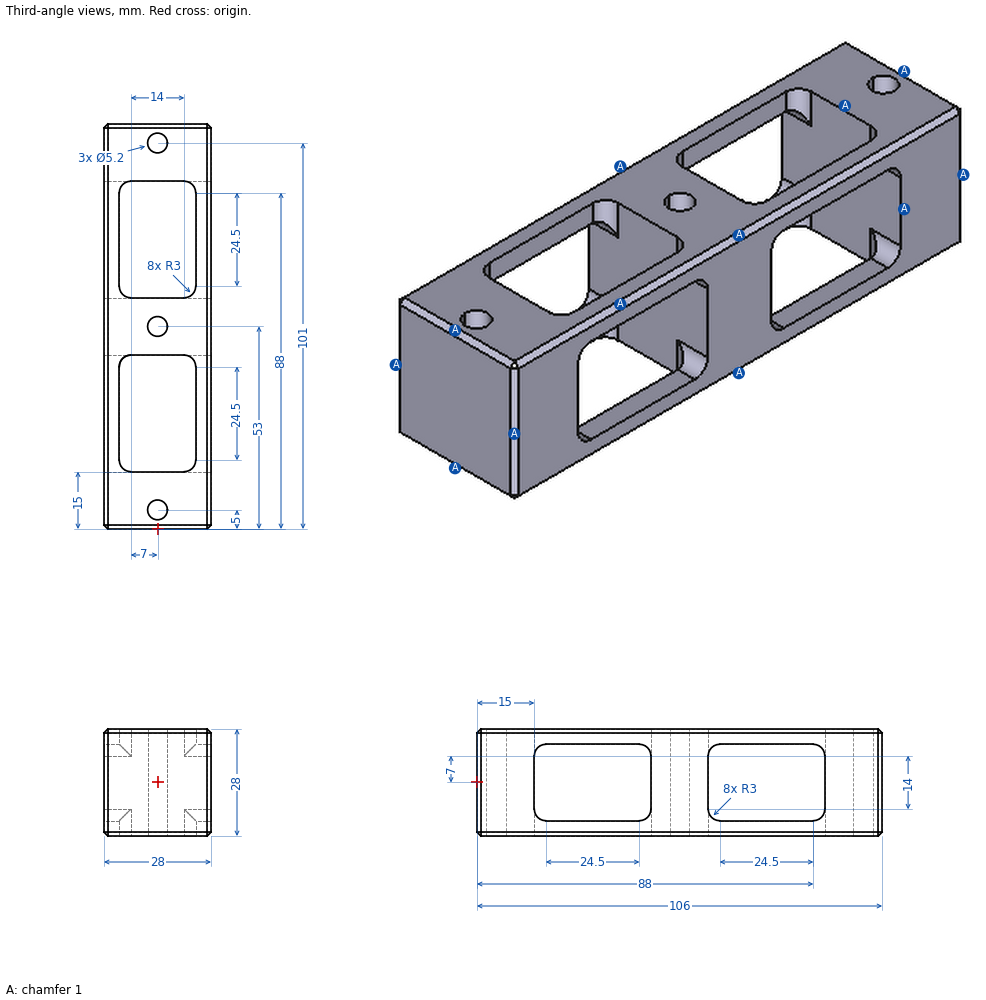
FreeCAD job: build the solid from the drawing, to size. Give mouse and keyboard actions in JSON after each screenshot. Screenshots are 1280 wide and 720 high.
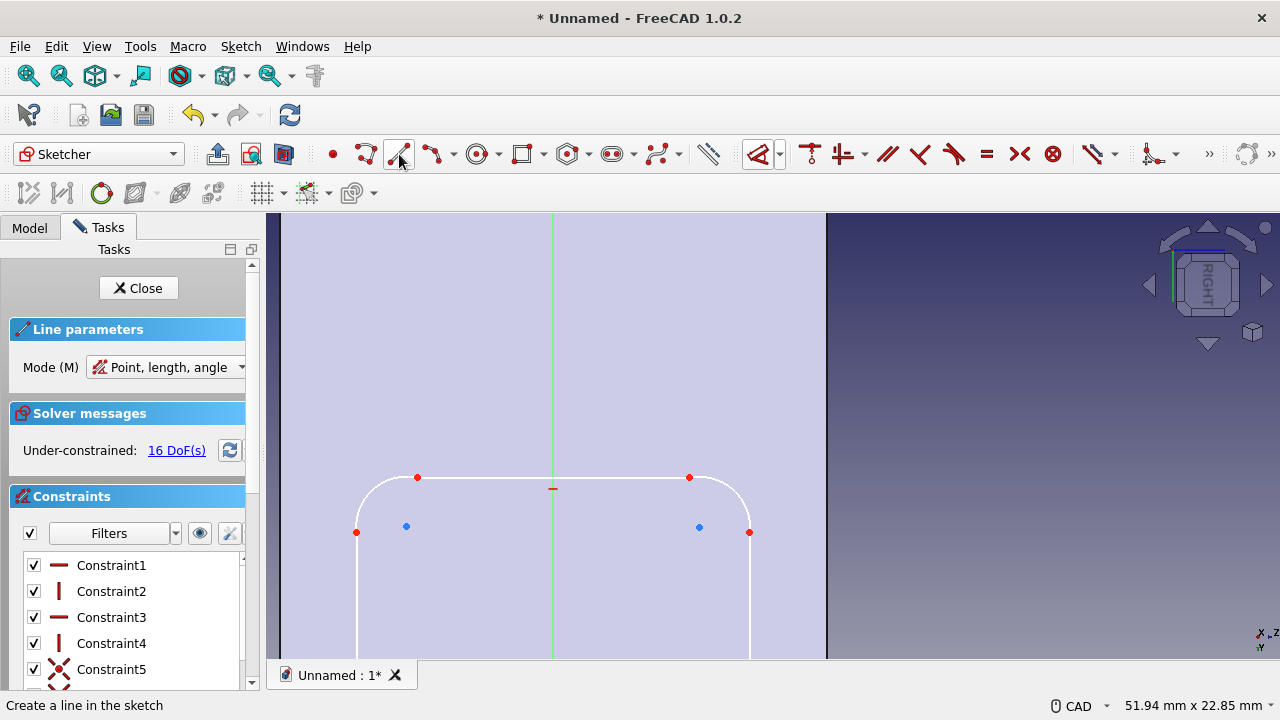
{"action": "scroll", "coordinate": [734, 487], "scroll_direction": "down", "scroll_amount": 9}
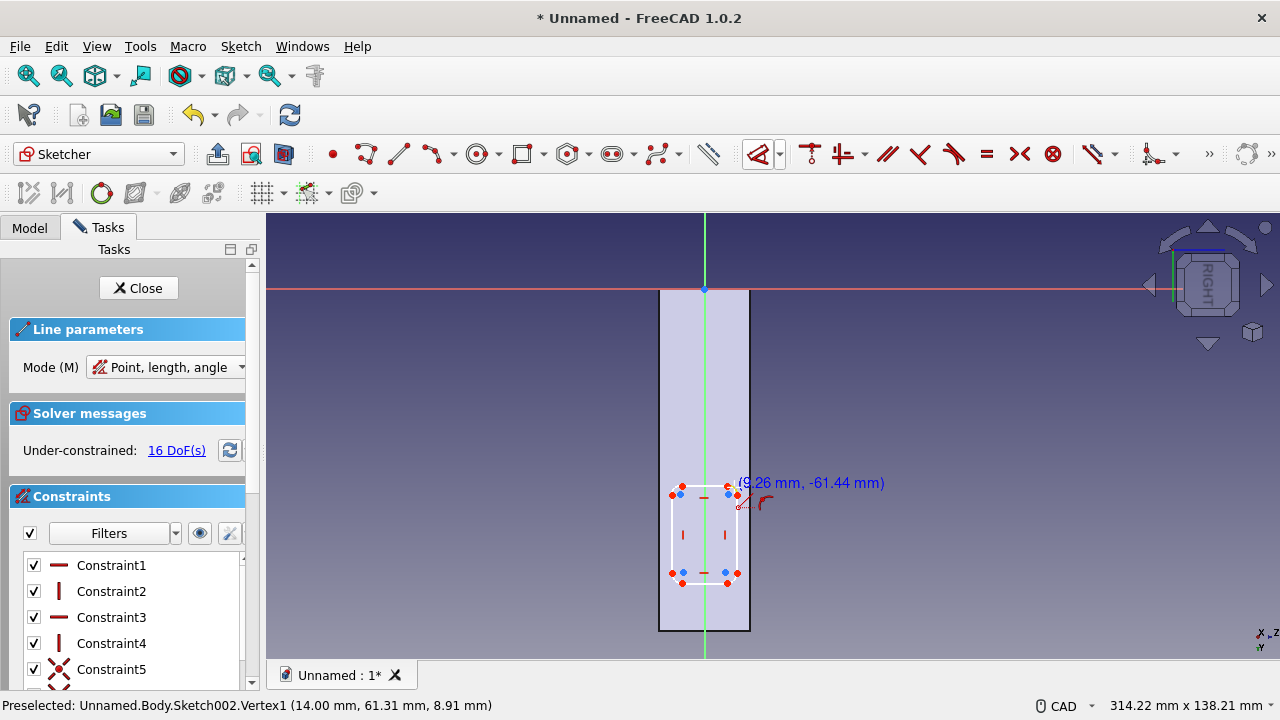
{"action": "left_click", "coordinate": [727, 338]}
{"action": "left_click", "coordinate": [682, 338]}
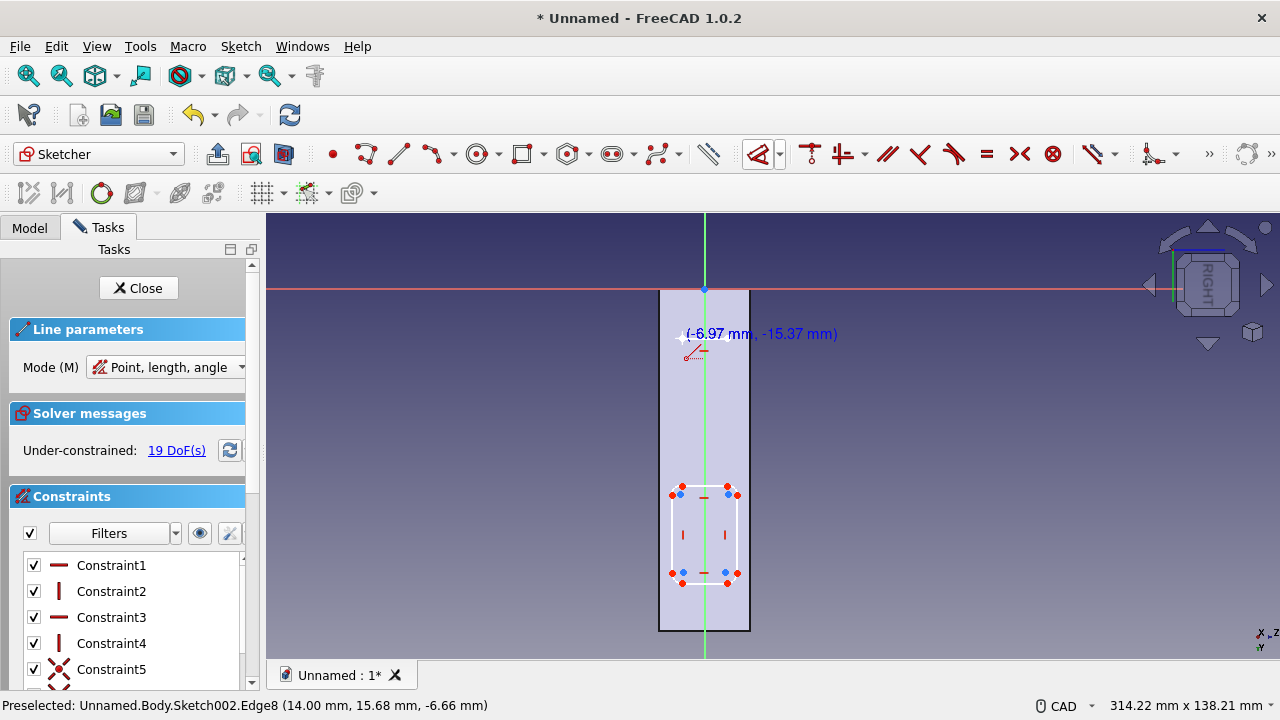
{"action": "left_click", "coordinate": [672, 347]}
{"action": "left_click", "coordinate": [672, 427]}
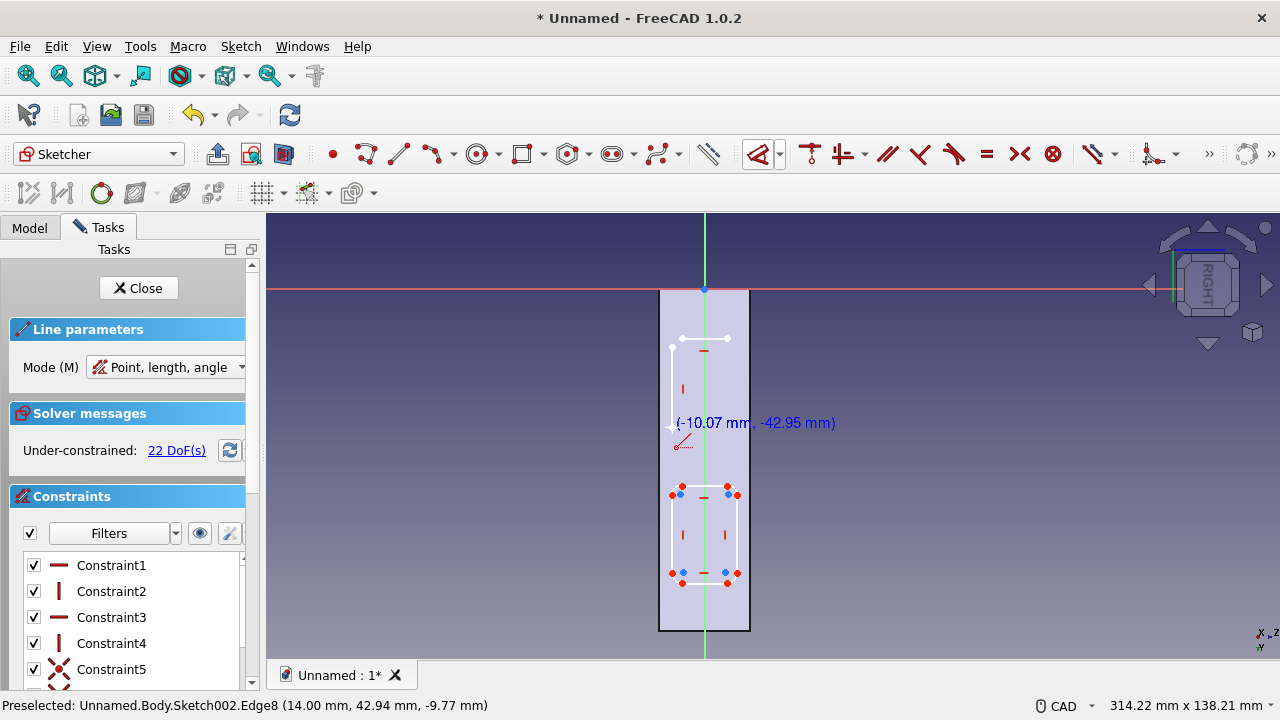
{"action": "left_click", "coordinate": [682, 436]}
{"action": "left_click", "coordinate": [727, 436]}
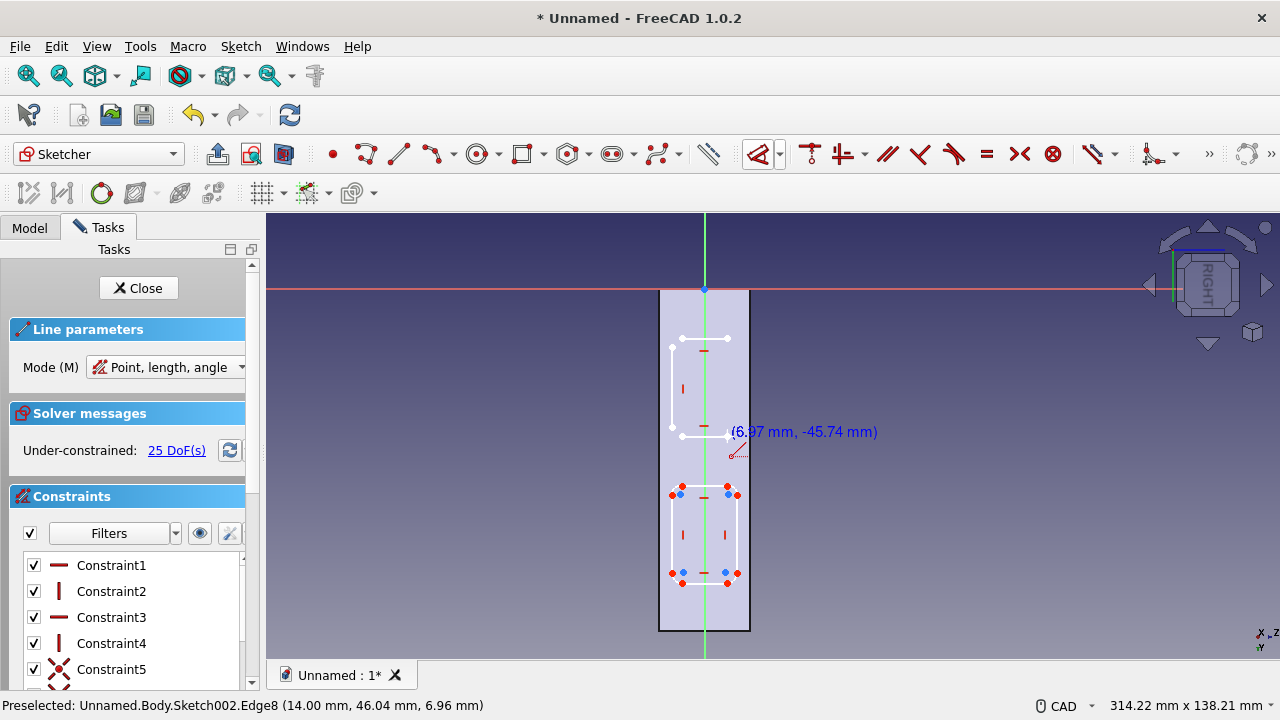
{"action": "left_click", "coordinate": [737, 427]}
{"action": "left_click", "coordinate": [737, 347]}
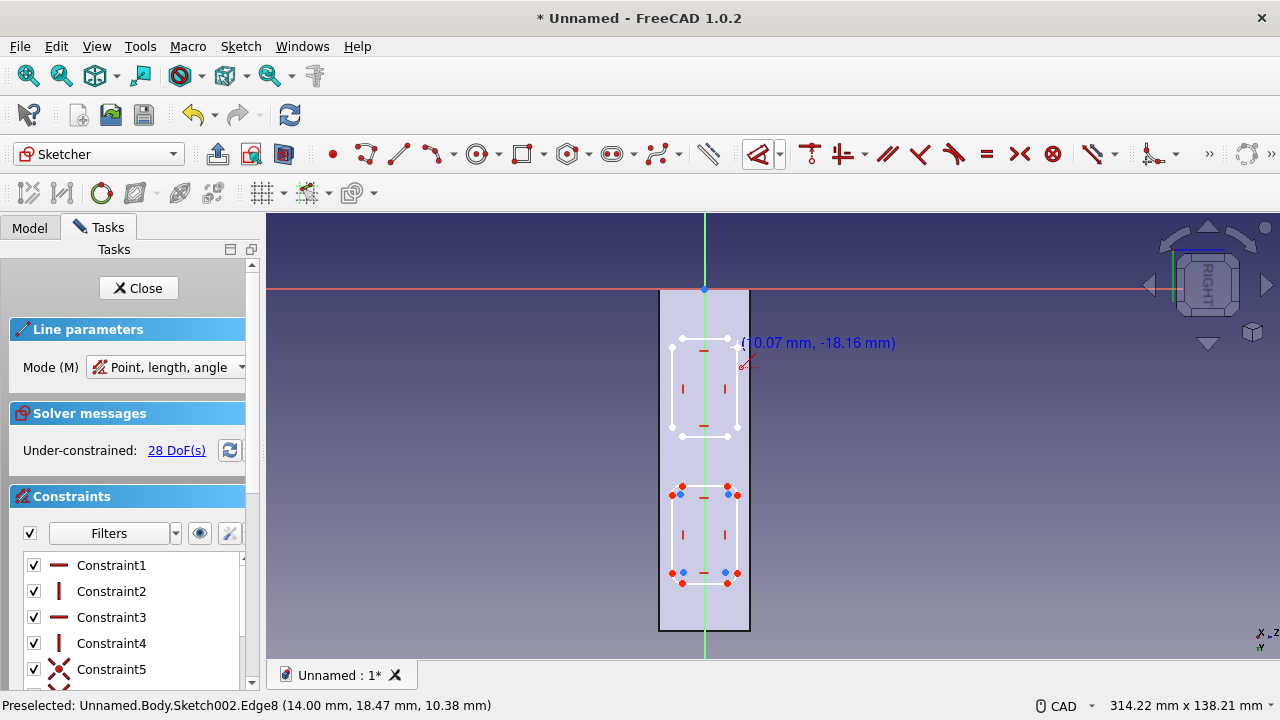
{"action": "left_click", "coordinate": [432, 154]}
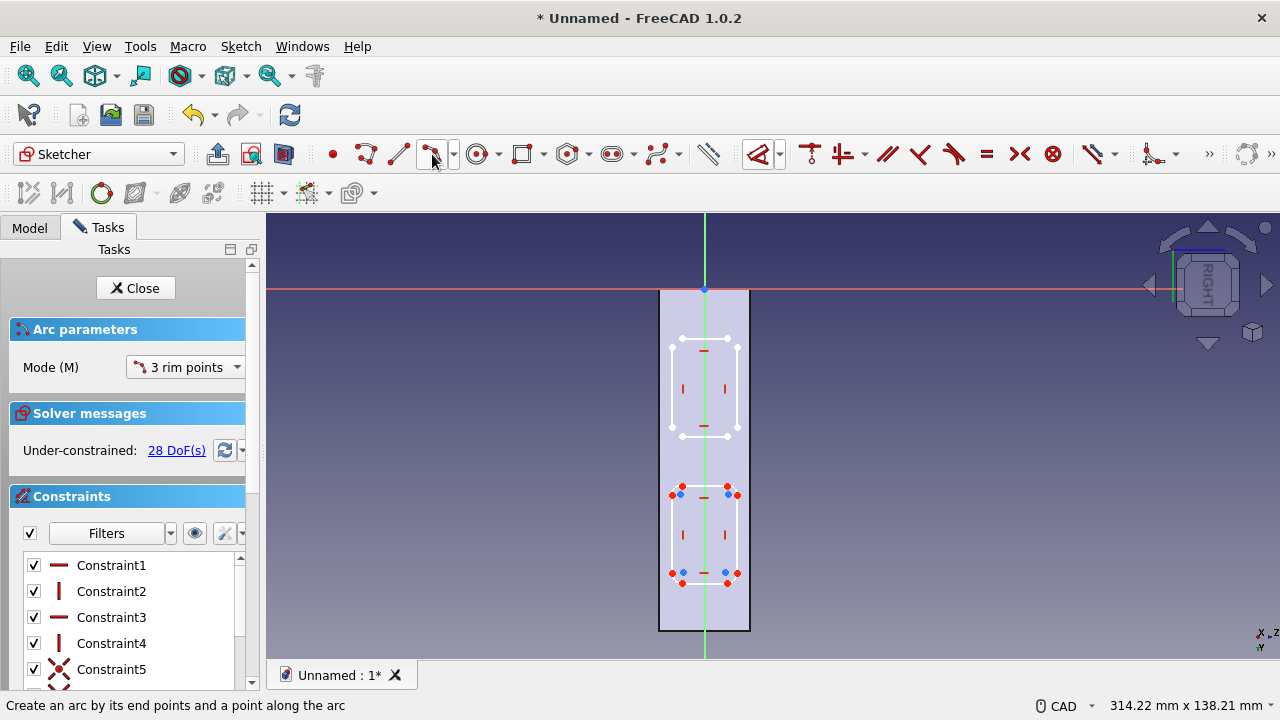
{"action": "left_click", "coordinate": [682, 339]}
{"action": "left_click", "coordinate": [672, 348]}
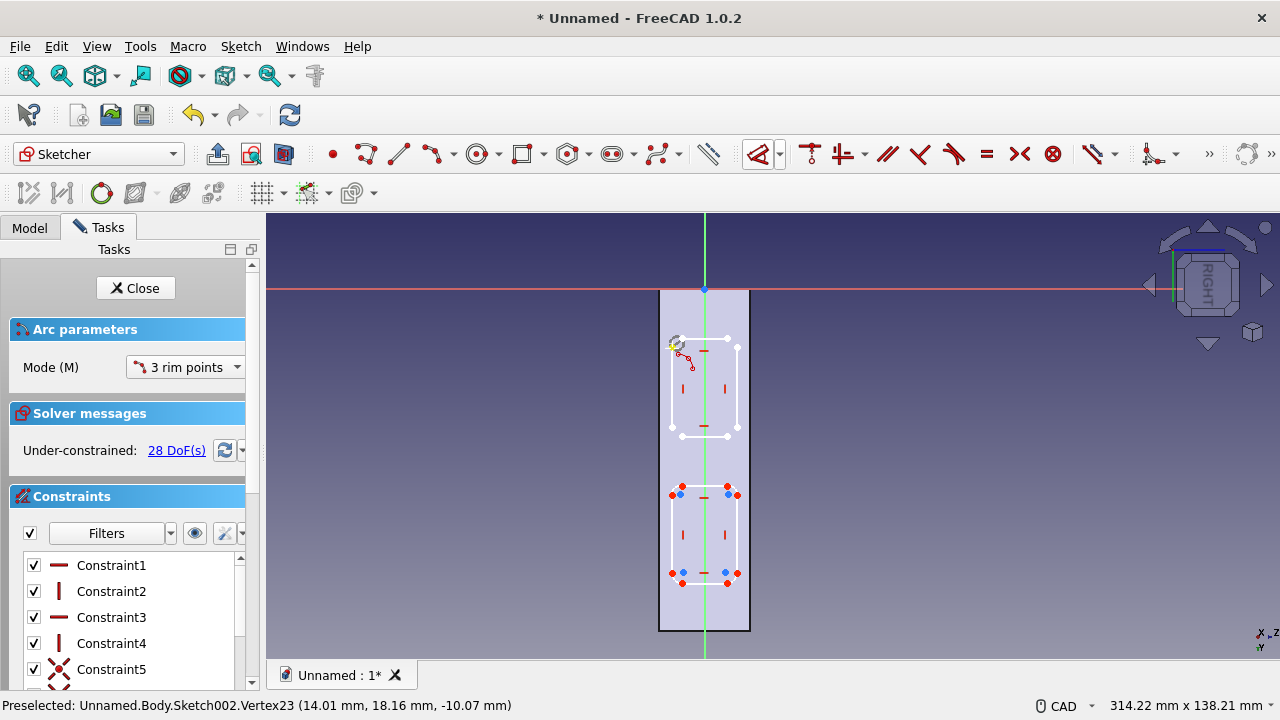
{"action": "scroll", "coordinate": [675, 341], "scroll_direction": "up", "scroll_amount": 9}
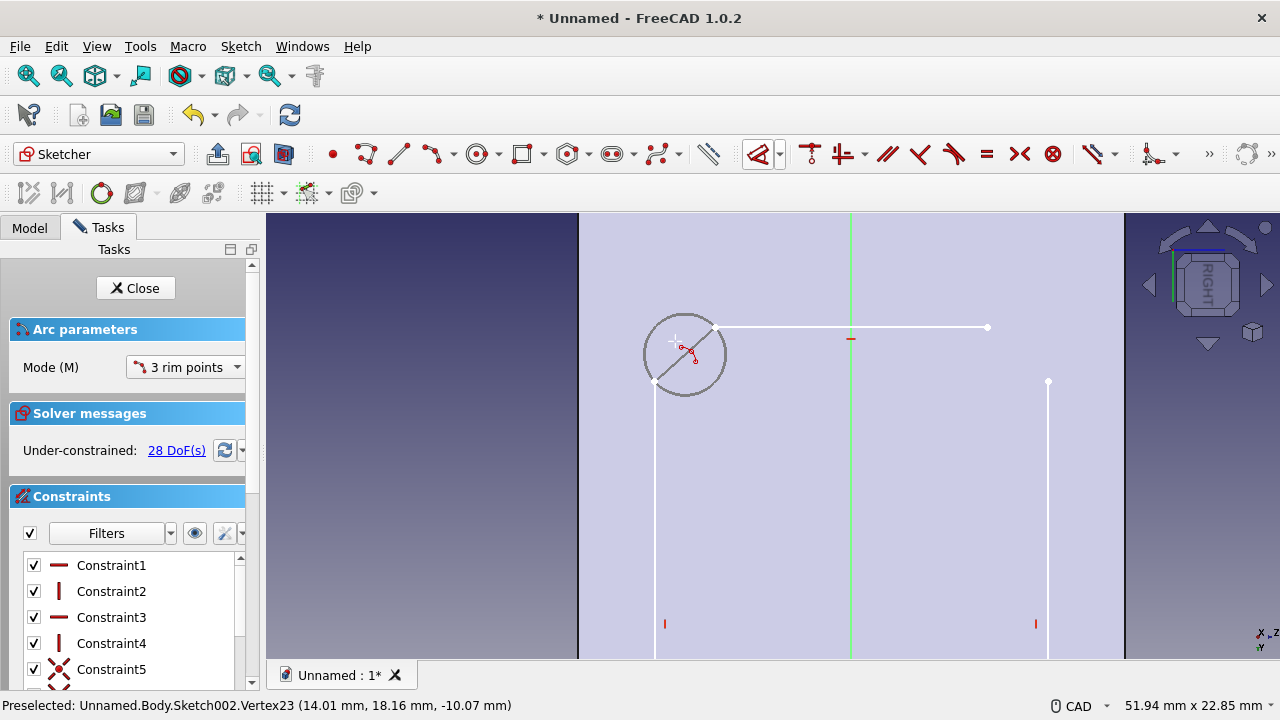
{"action": "left_click", "coordinate": [673, 337]}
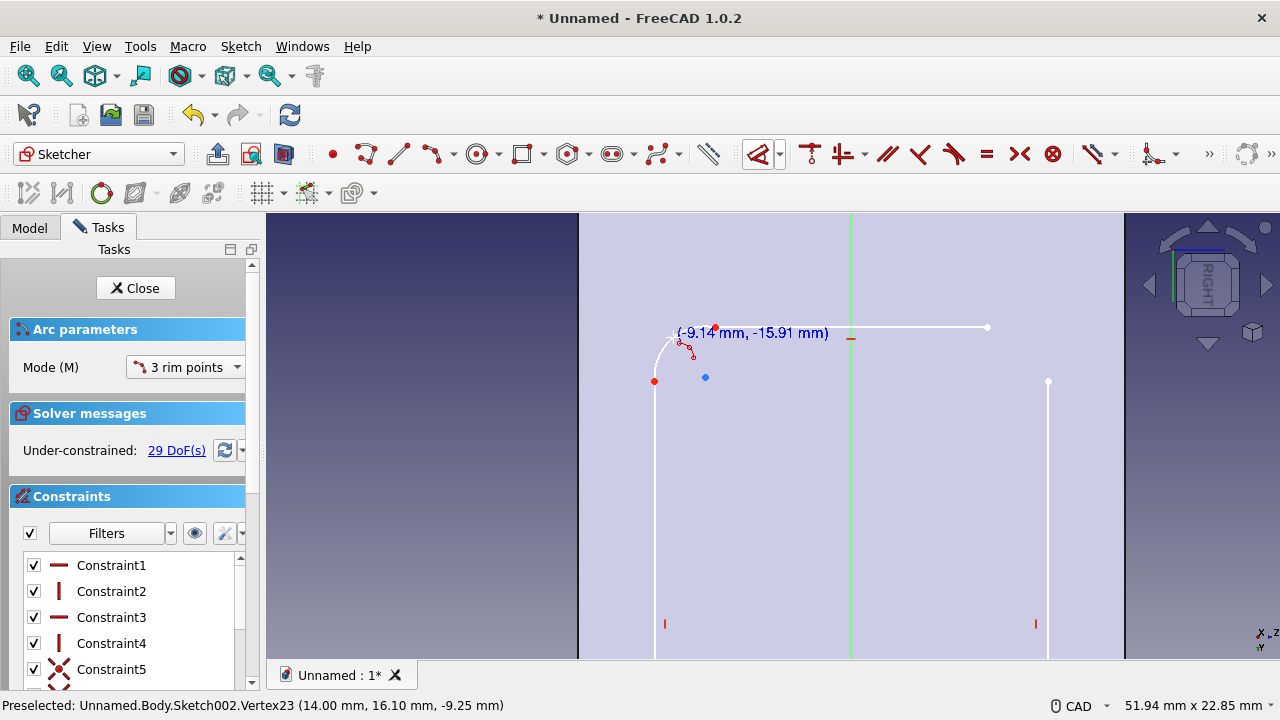
{"action": "scroll", "coordinate": [675, 341], "scroll_direction": "down", "scroll_amount": 9}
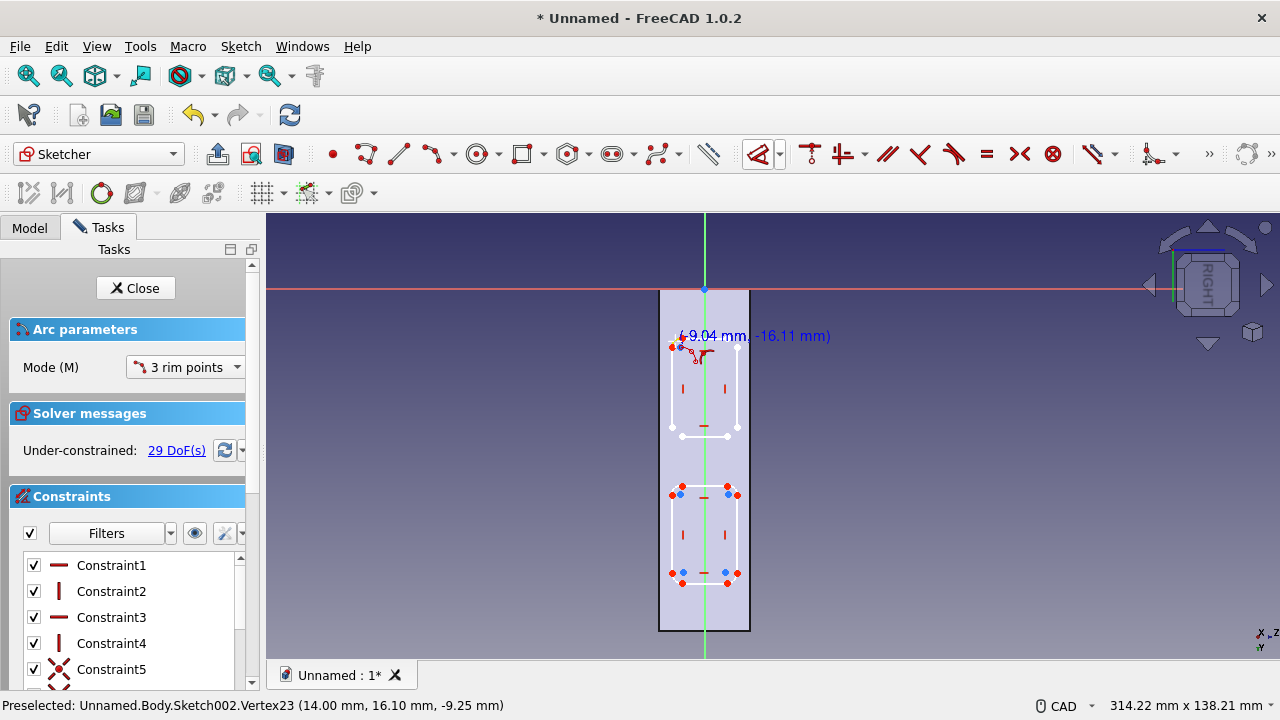
{"action": "left_click", "coordinate": [672, 428]}
{"action": "left_click", "coordinate": [682, 437]}